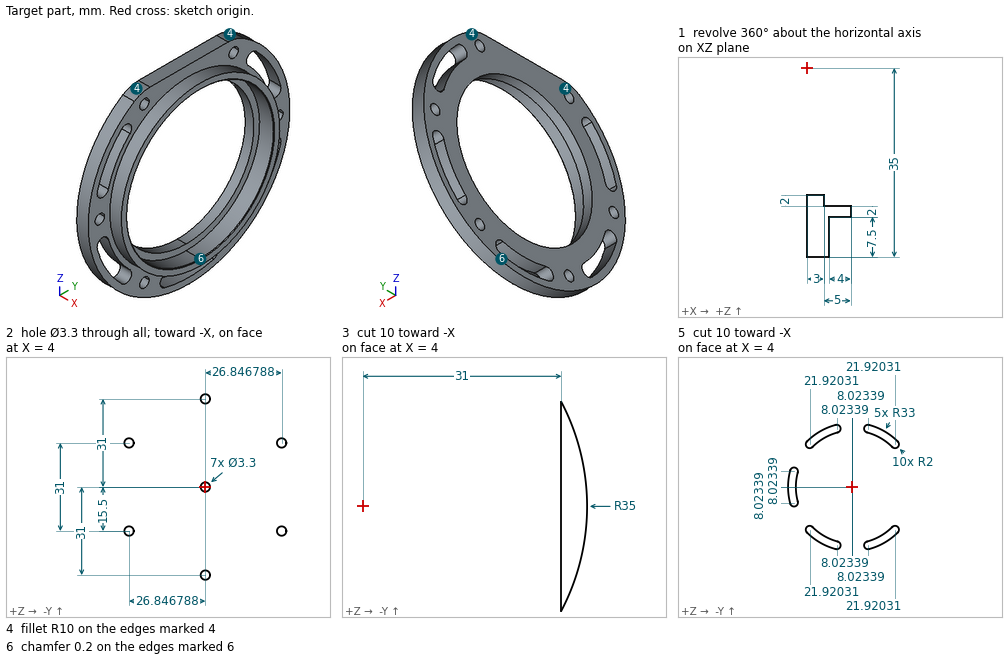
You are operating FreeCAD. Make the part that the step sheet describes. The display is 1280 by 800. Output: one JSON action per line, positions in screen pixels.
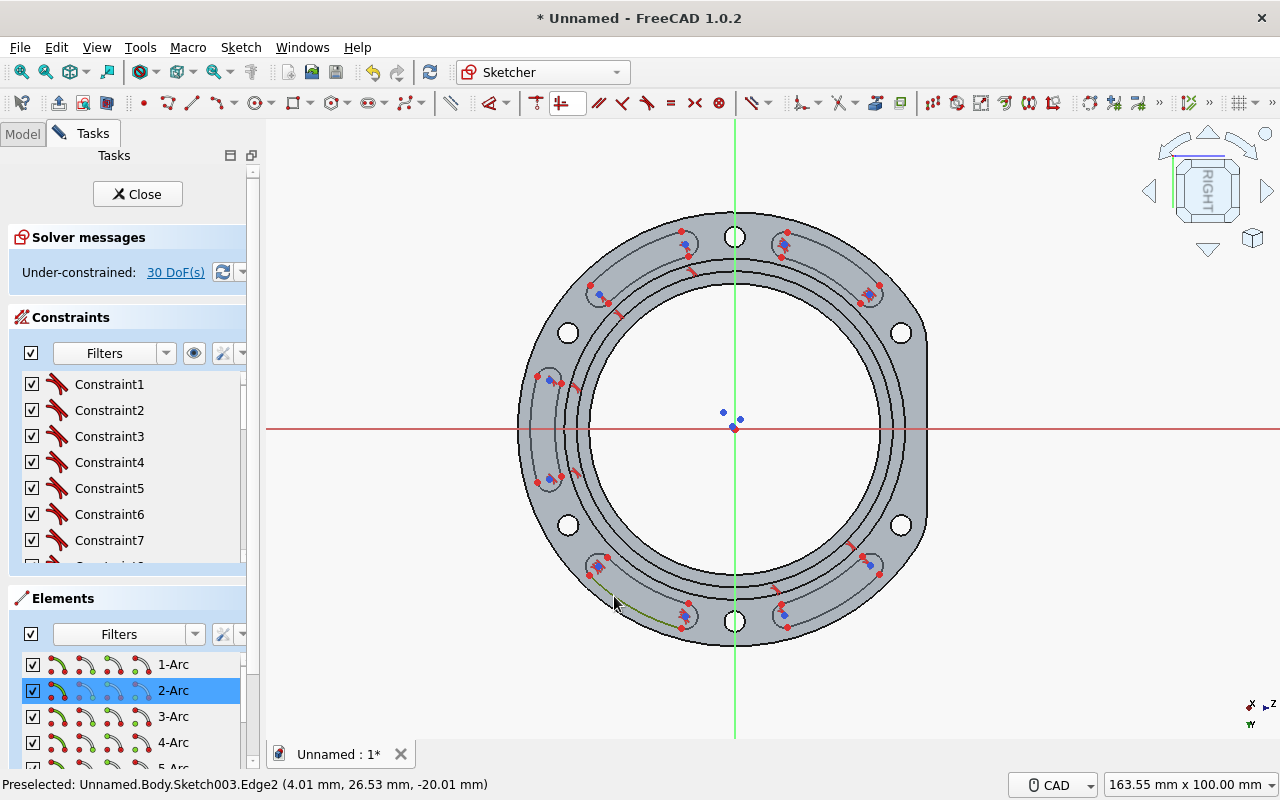
{"action": "left_click", "coordinate": [855, 264]}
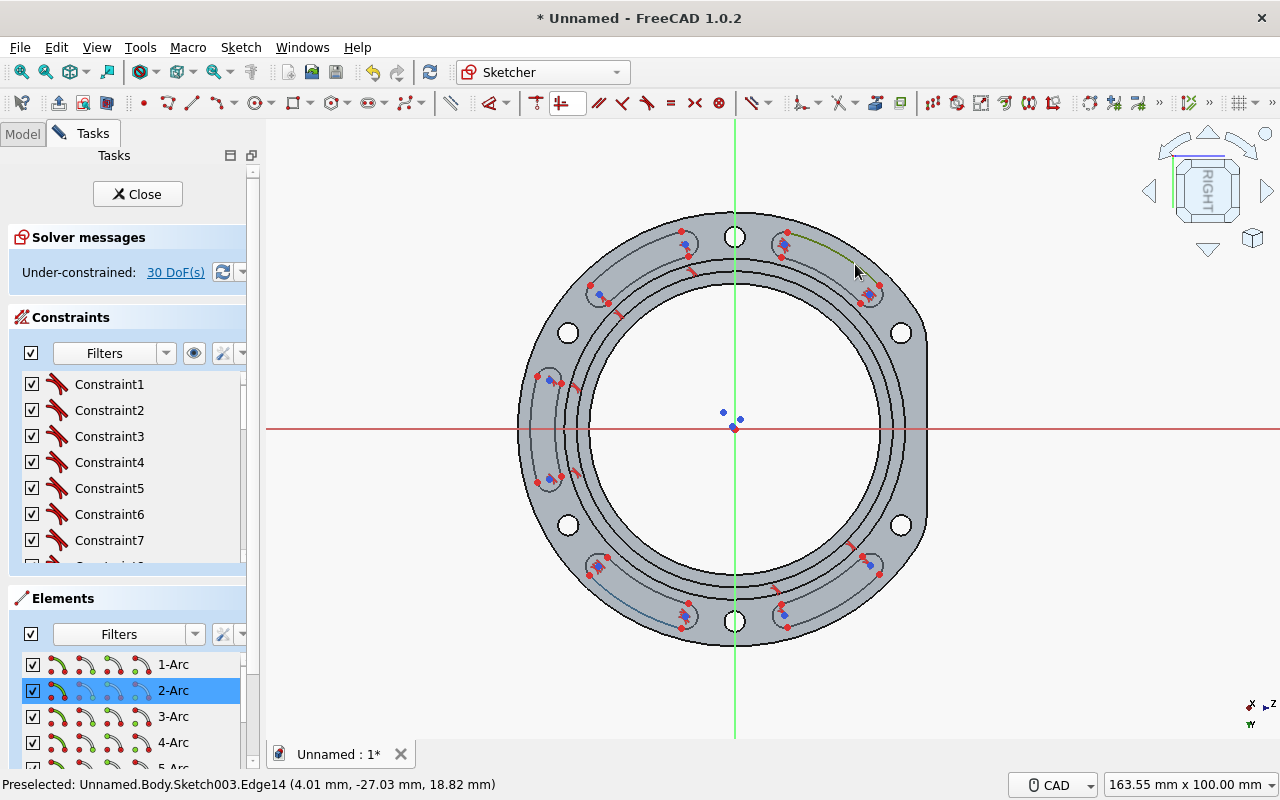
{"action": "left_click", "coordinate": [536, 104]}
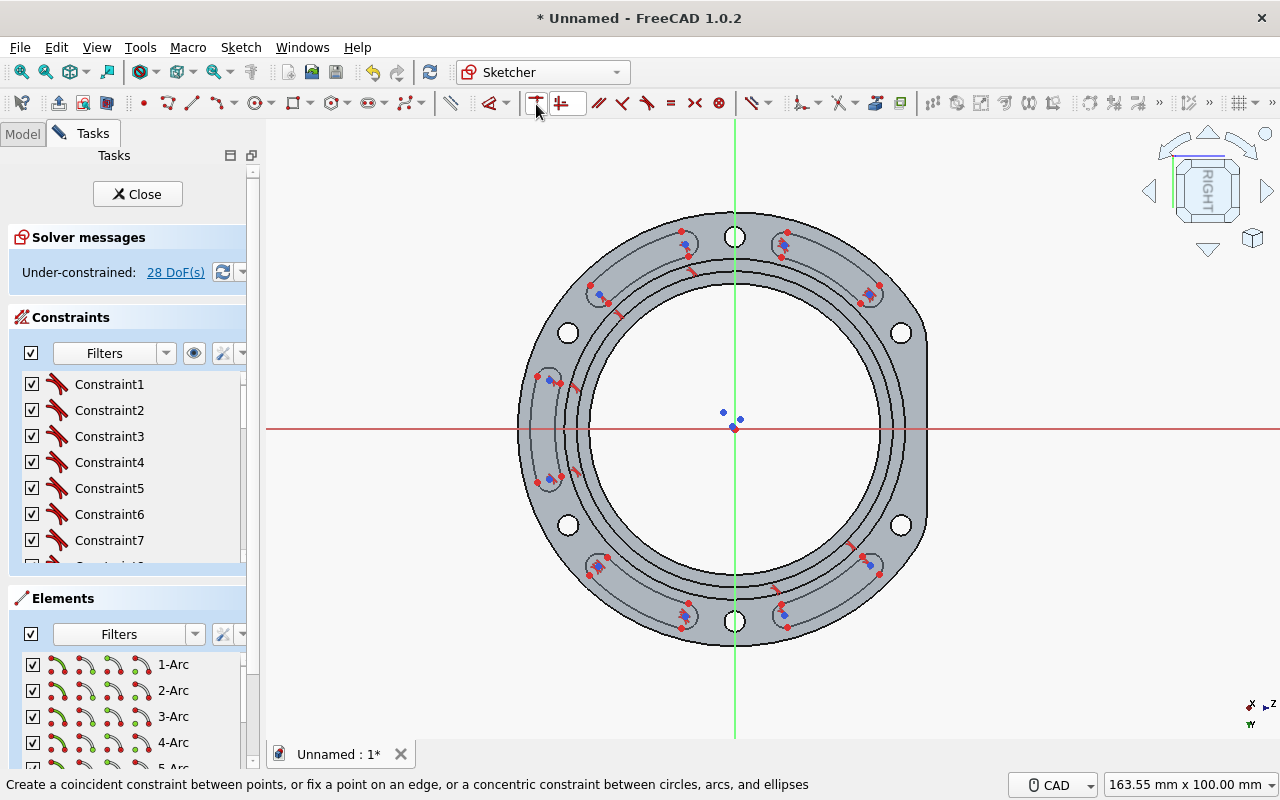
{"action": "left_click", "coordinate": [614, 596]}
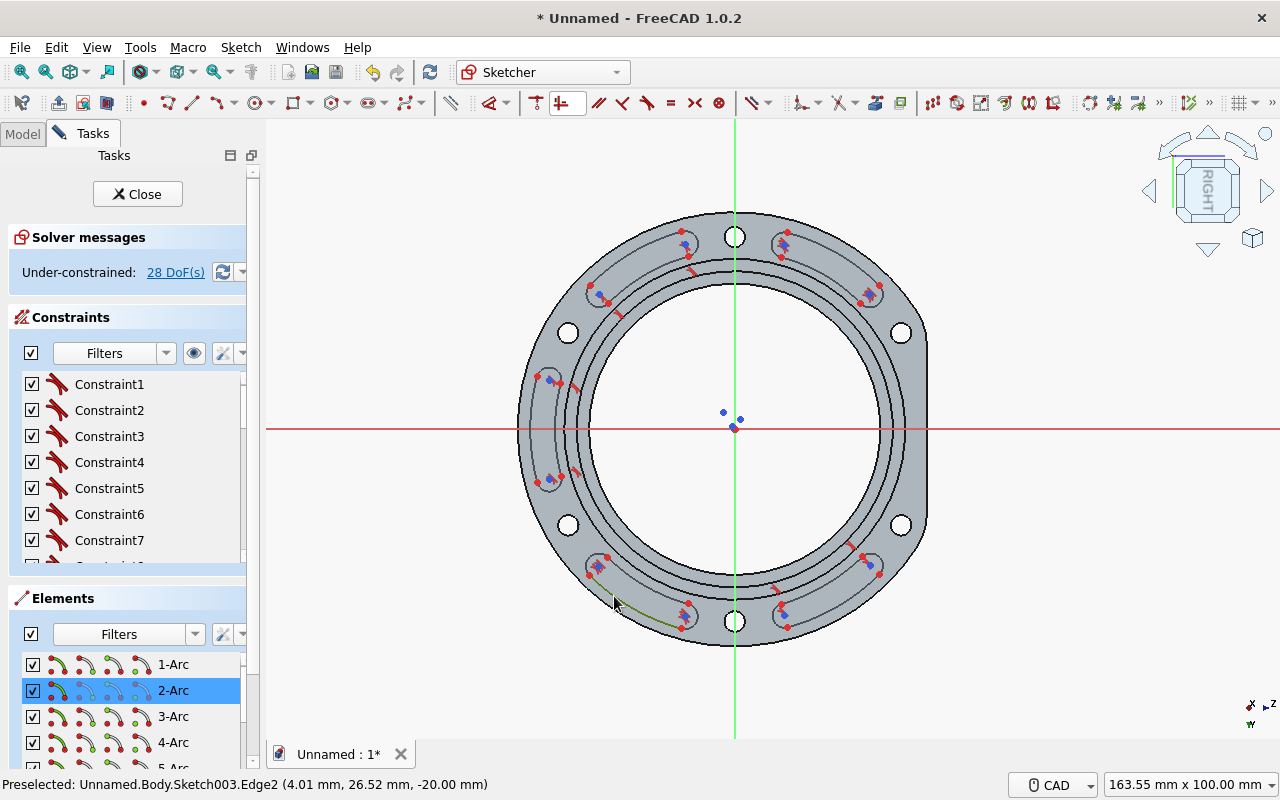
{"action": "left_click", "coordinate": [840, 285]}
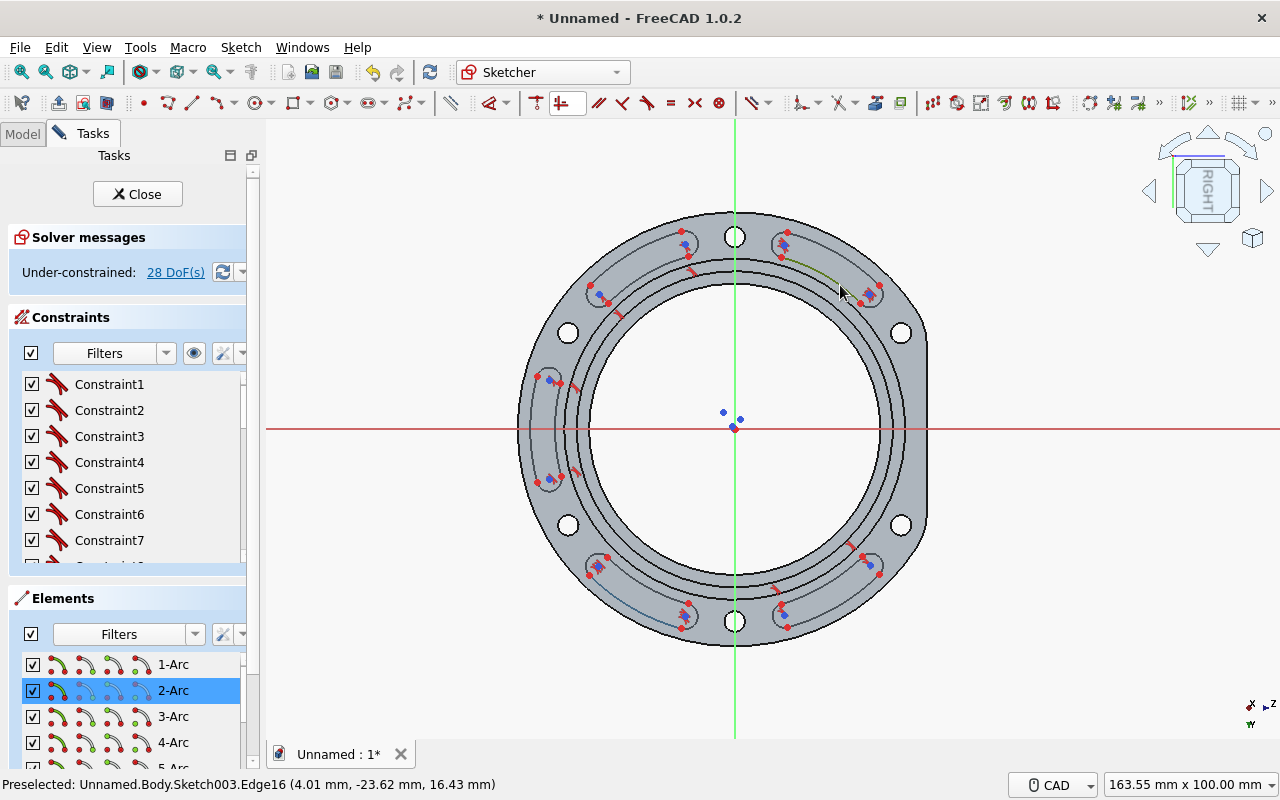
{"action": "left_click", "coordinate": [536, 104]}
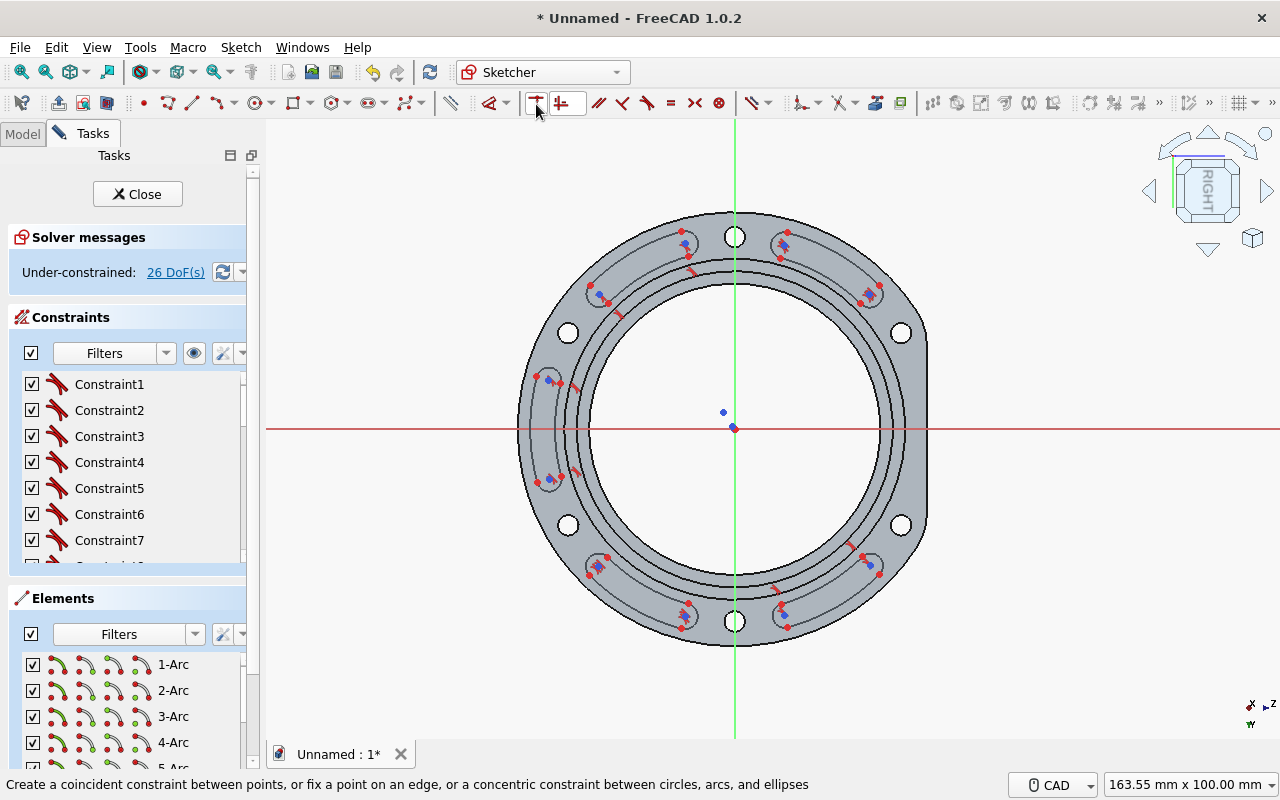
{"action": "left_click", "coordinate": [614, 596]}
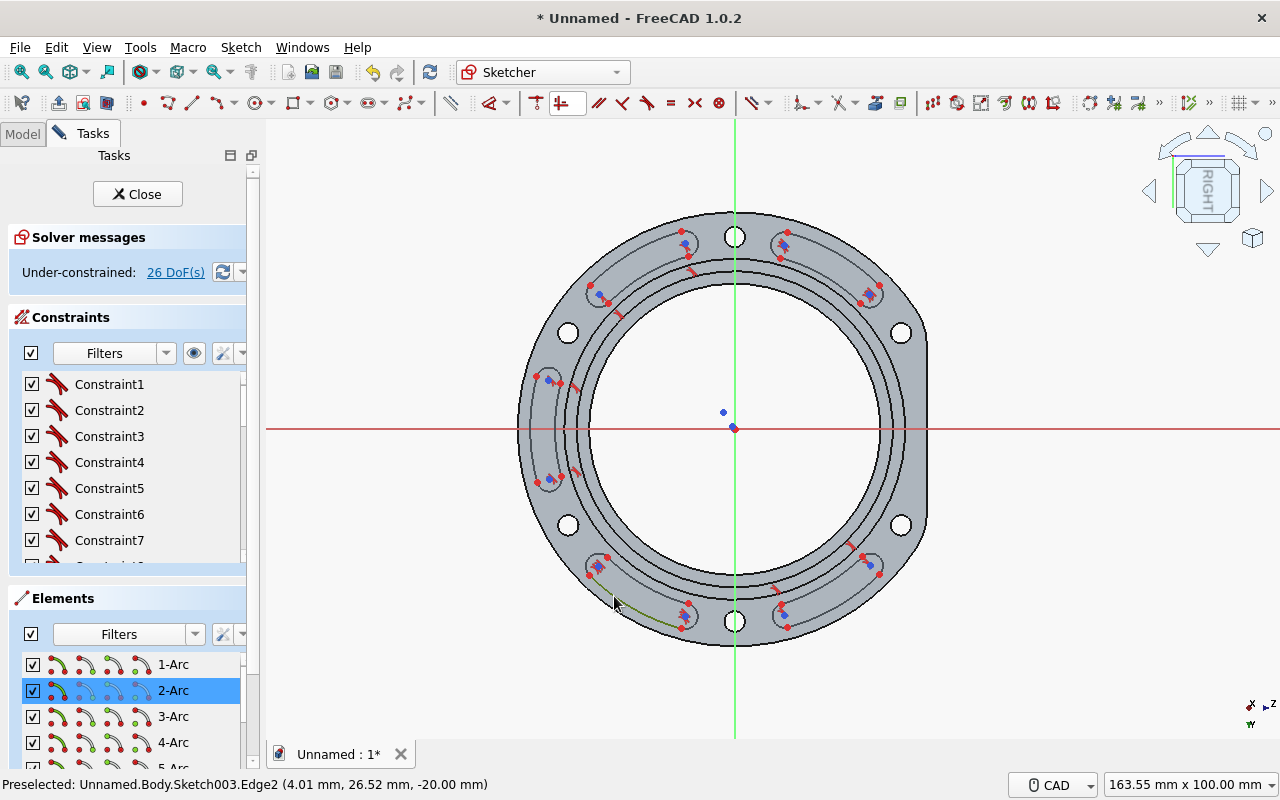
{"action": "left_click", "coordinate": [808, 594]}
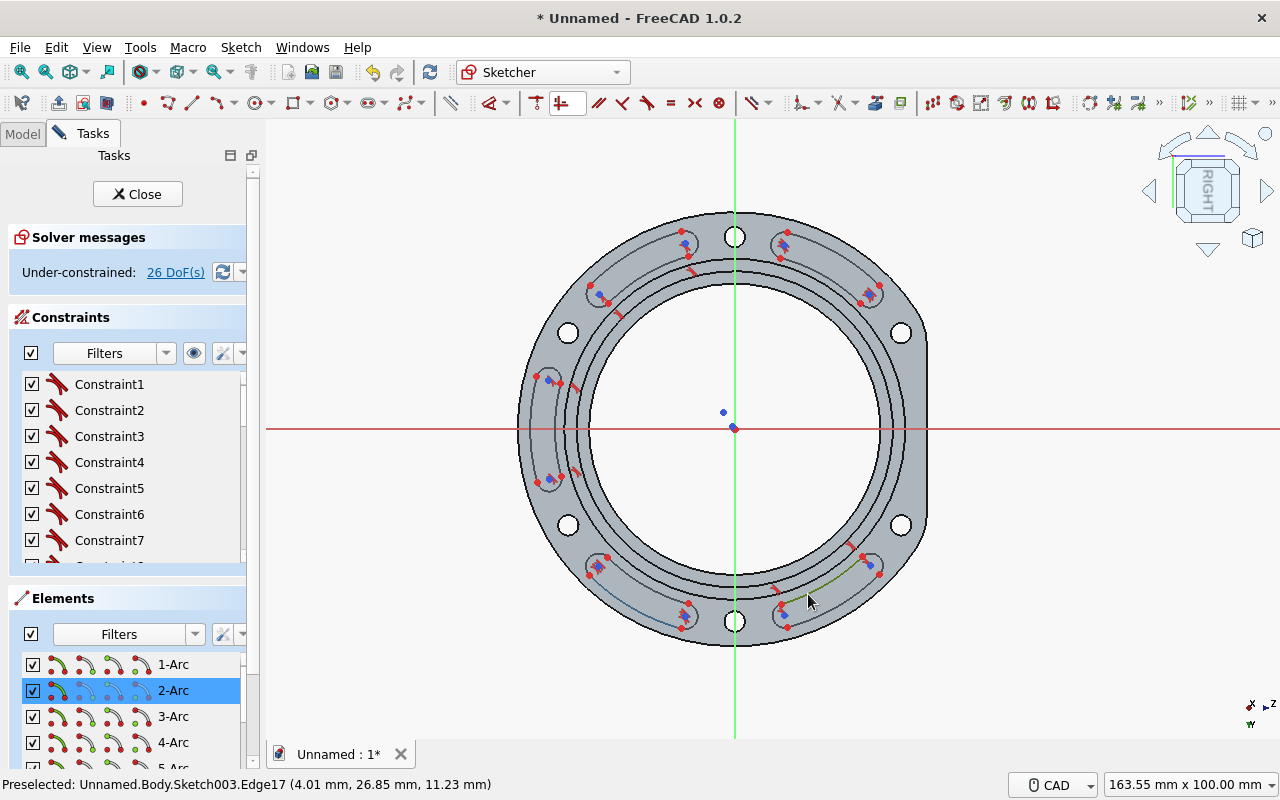
{"action": "left_click", "coordinate": [536, 104]}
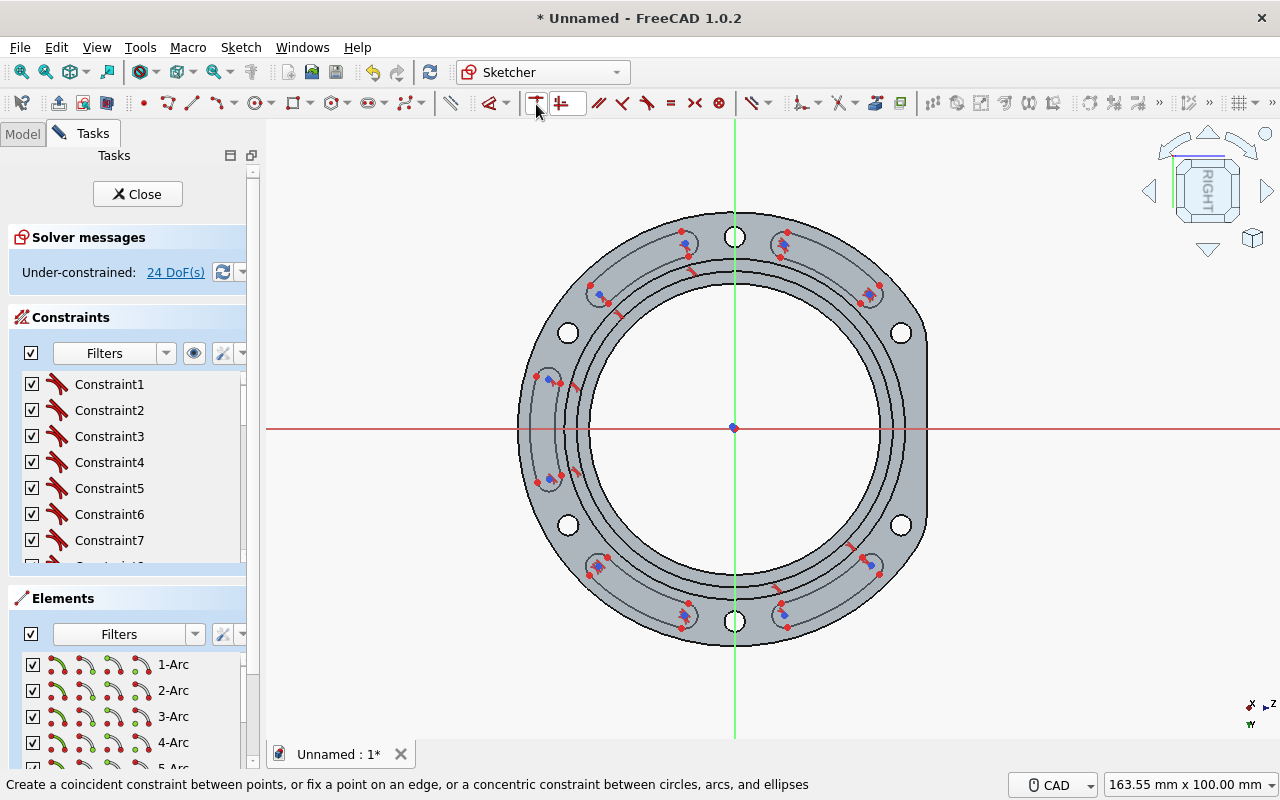
{"action": "left_click", "coordinate": [614, 596]}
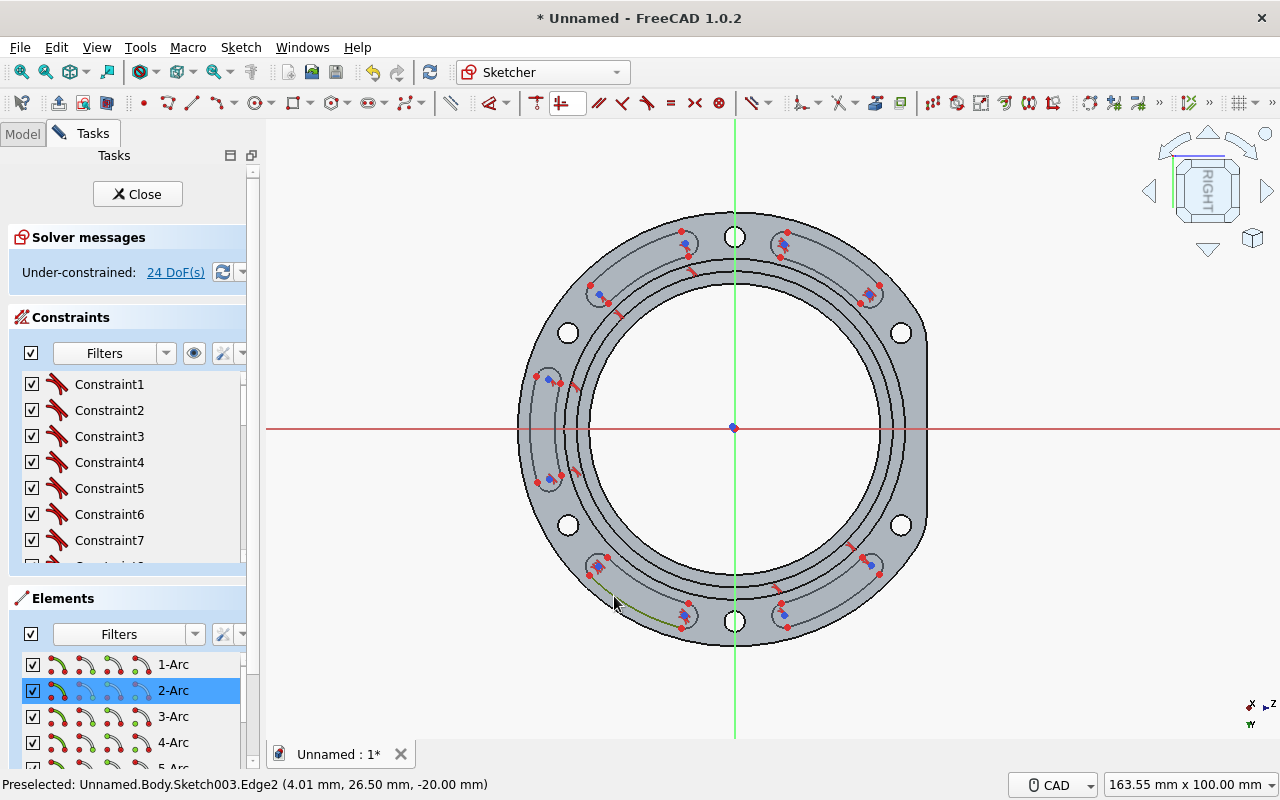
{"action": "left_click", "coordinate": [818, 617]}